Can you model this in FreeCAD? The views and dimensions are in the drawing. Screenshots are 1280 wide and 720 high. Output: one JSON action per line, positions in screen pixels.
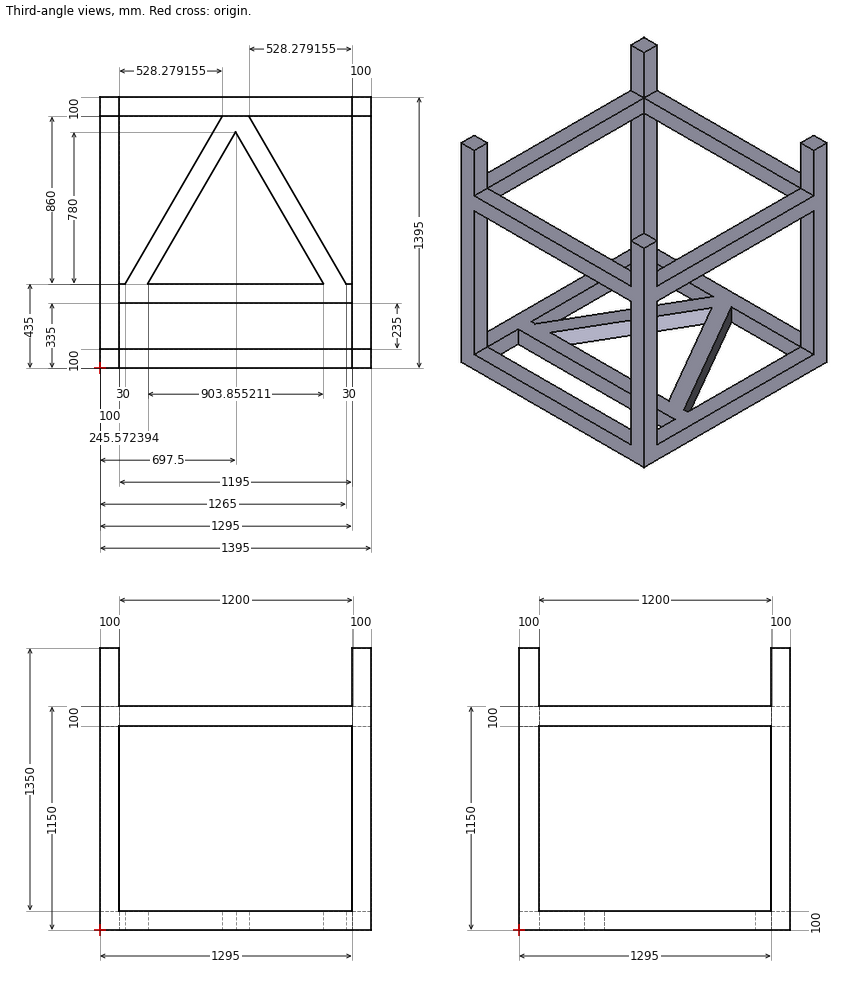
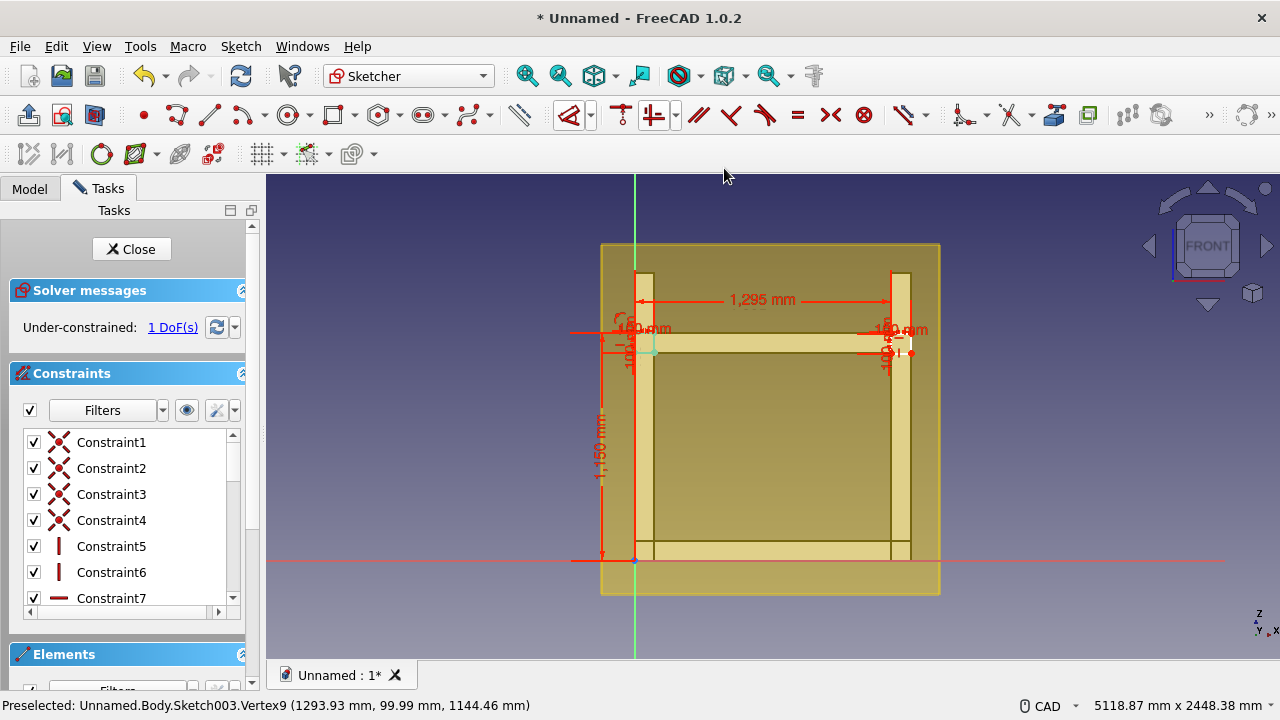
{"action": "left_click", "coordinate": [891, 334]}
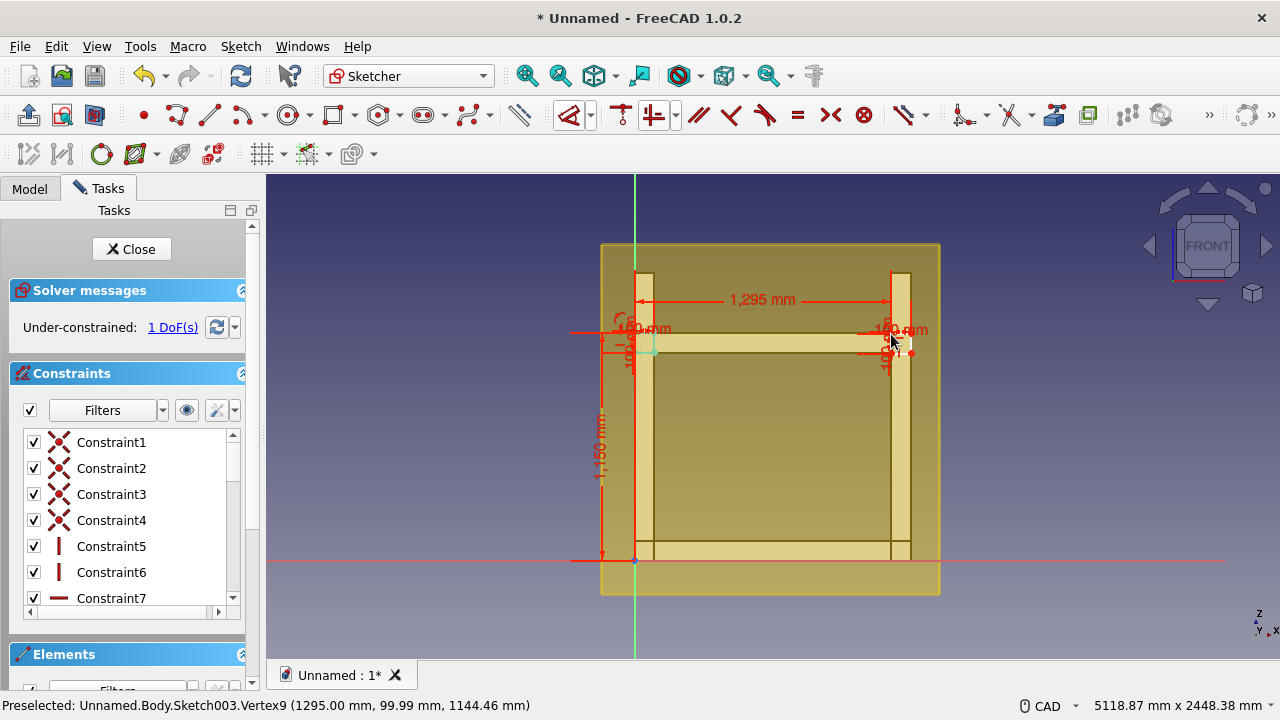
{"action": "key", "text": "i"}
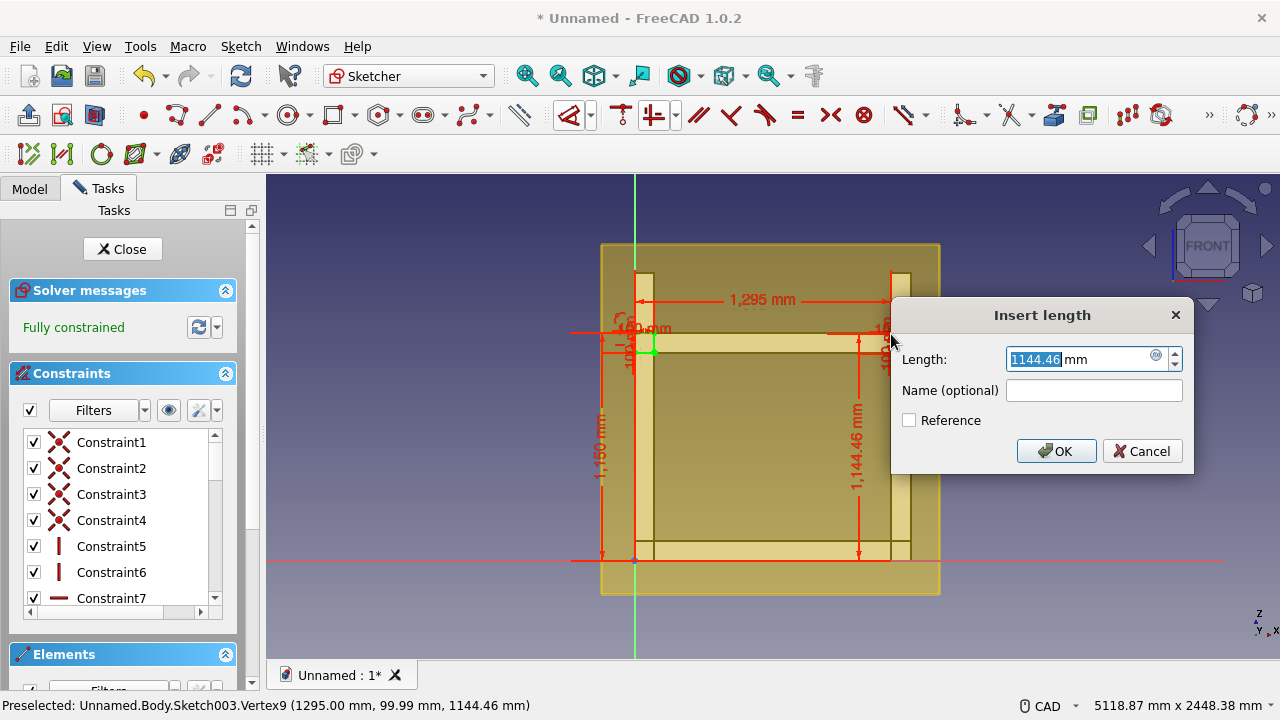
{"action": "type", "text": "1150"}
{"action": "key", "text": "Return"}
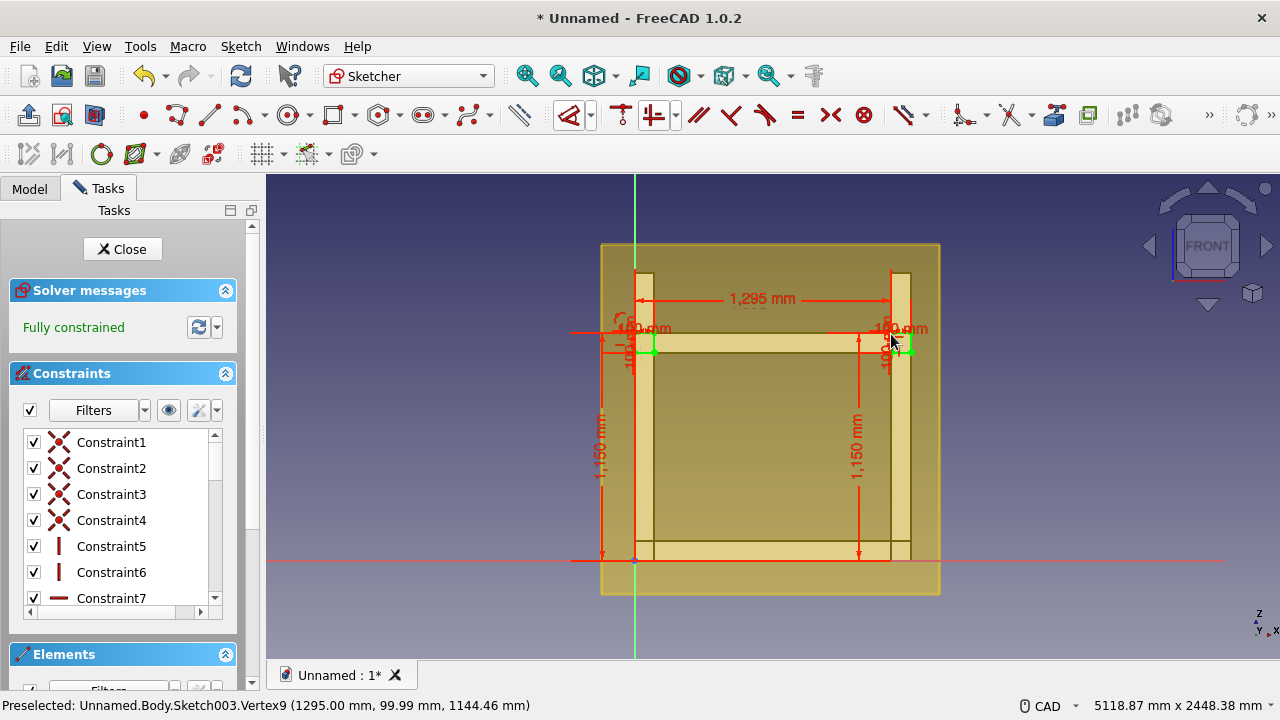
{"action": "left_click", "coordinate": [123, 249]}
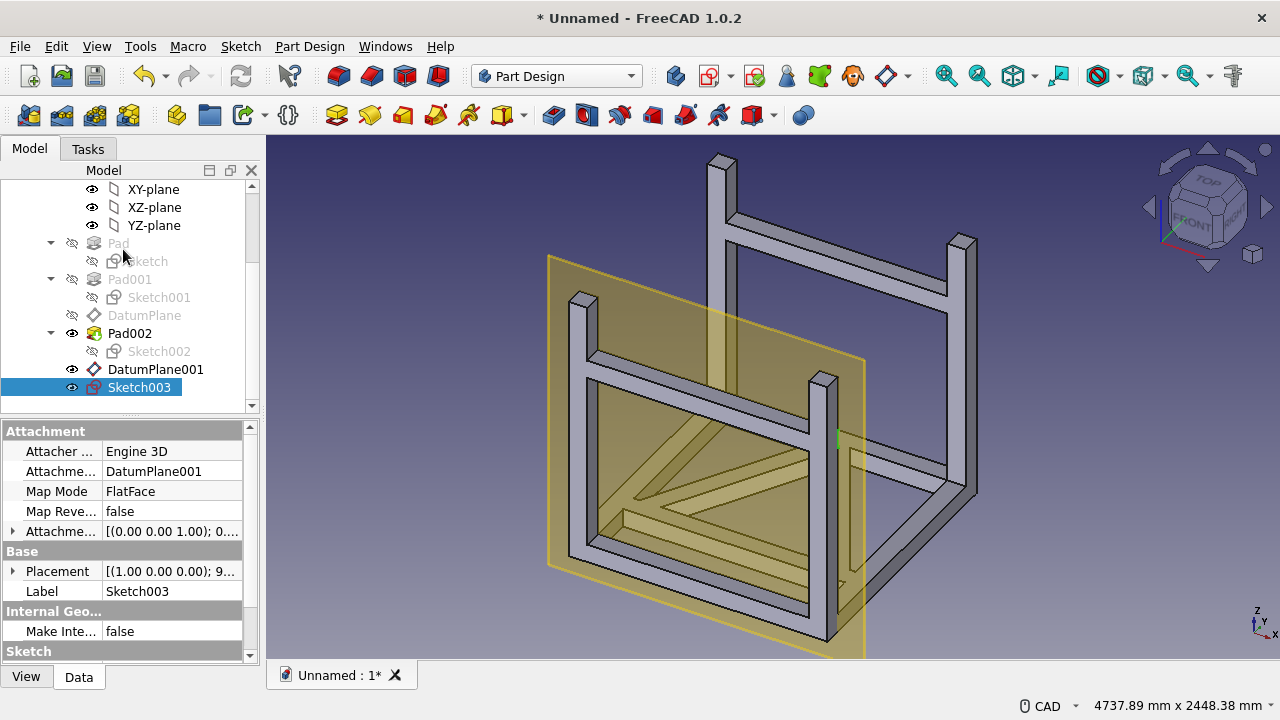
{"action": "left_click", "coordinate": [337, 116]}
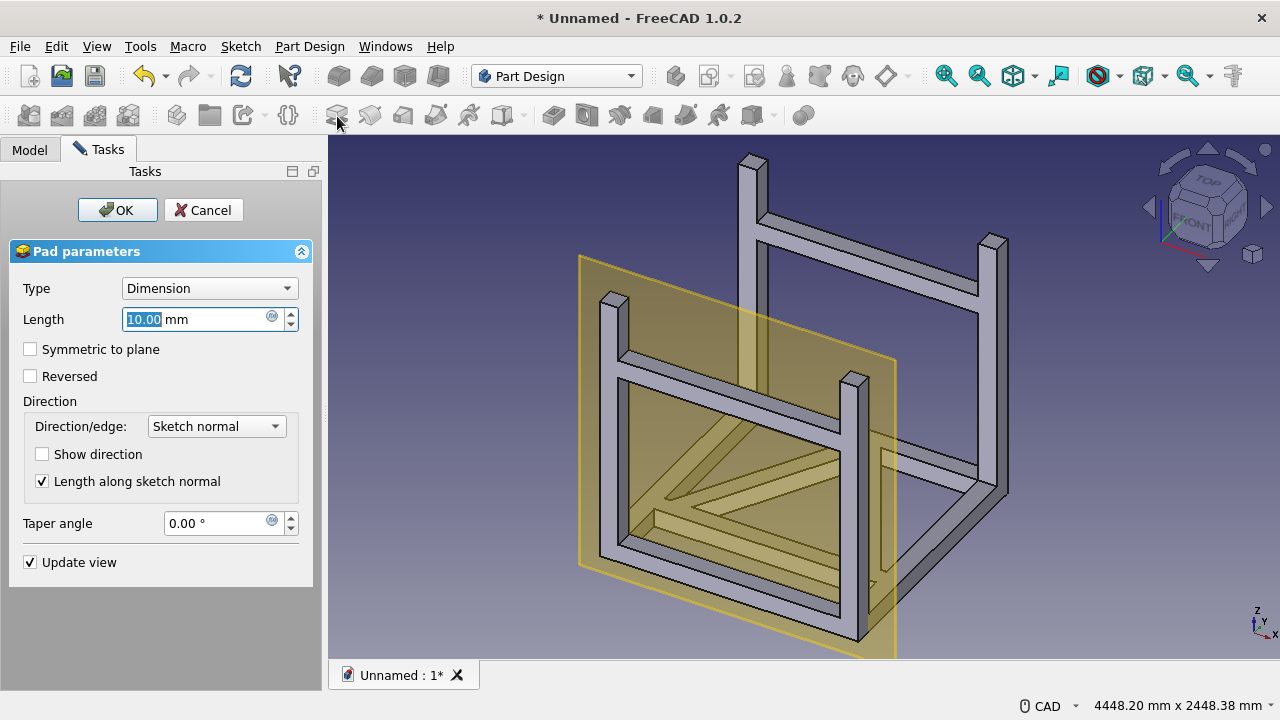
{"action": "type", "text": "1200"}
{"action": "key", "text": "Tab"}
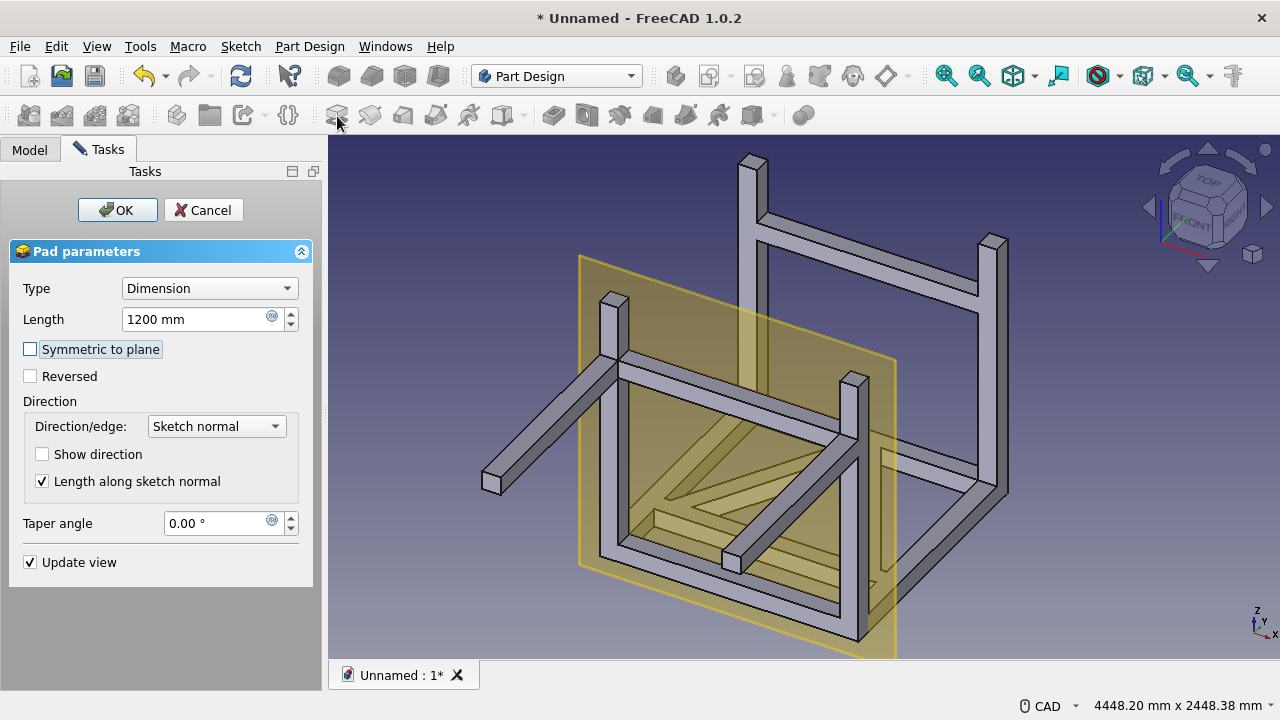
{"action": "left_click", "coordinate": [31, 376]}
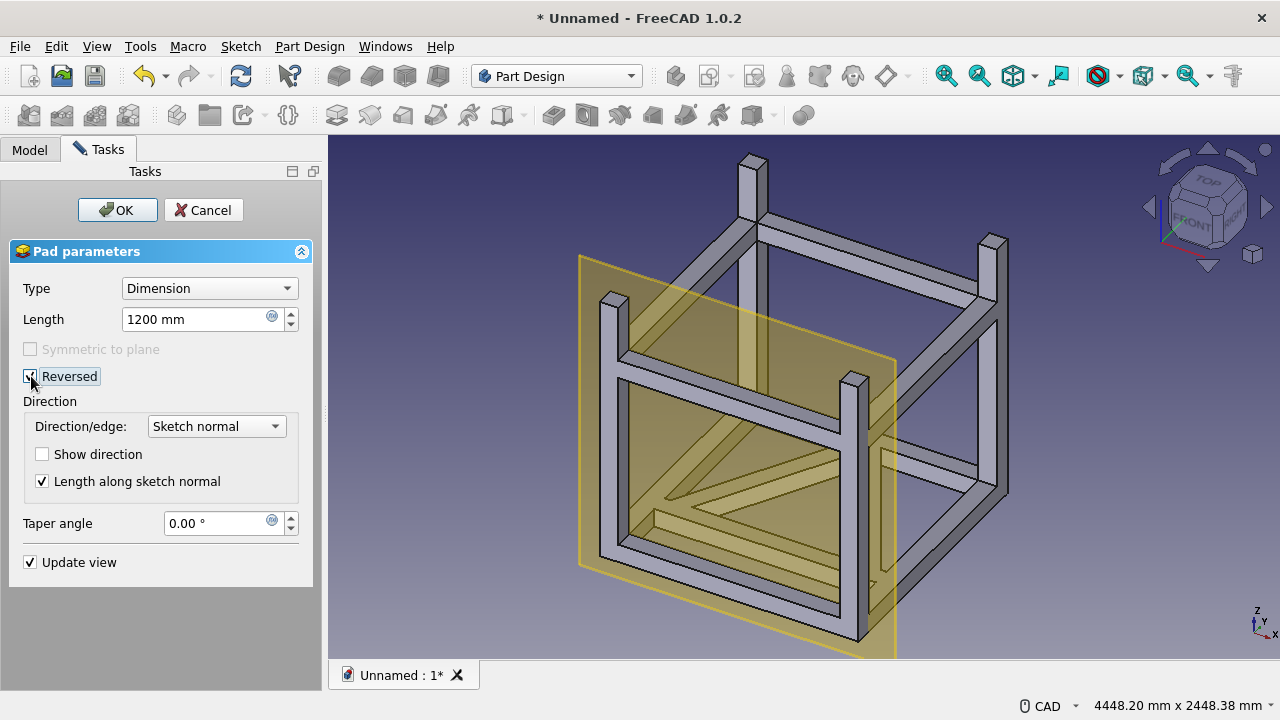
{"action": "left_click", "coordinate": [118, 210]}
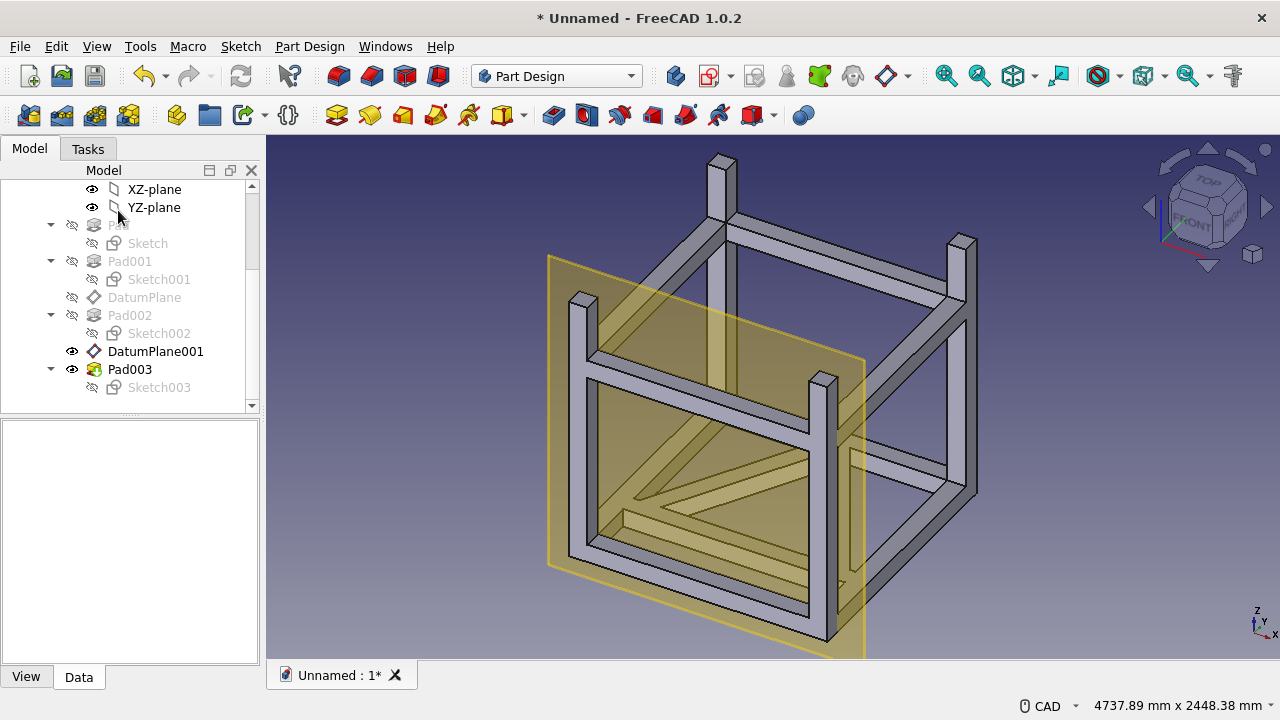
{"action": "left_click", "coordinate": [117, 351]}
{"action": "key", "text": "space"}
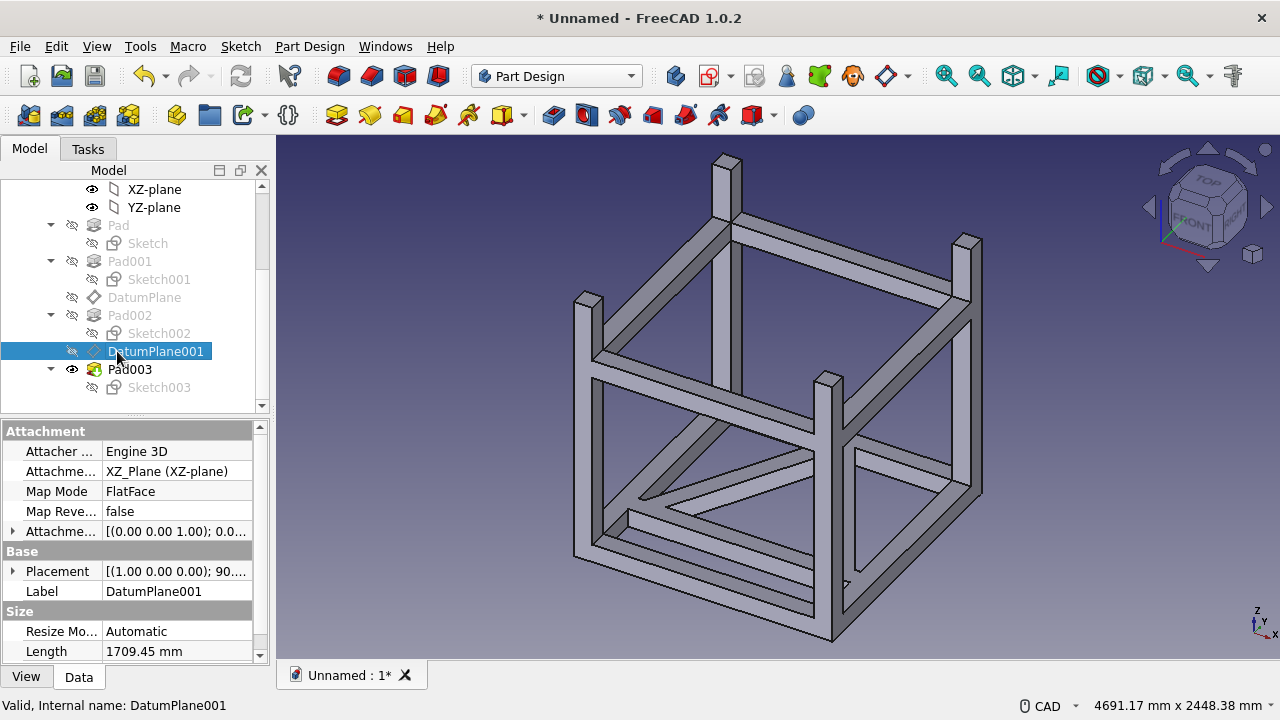
{"action": "key", "text": "0"}